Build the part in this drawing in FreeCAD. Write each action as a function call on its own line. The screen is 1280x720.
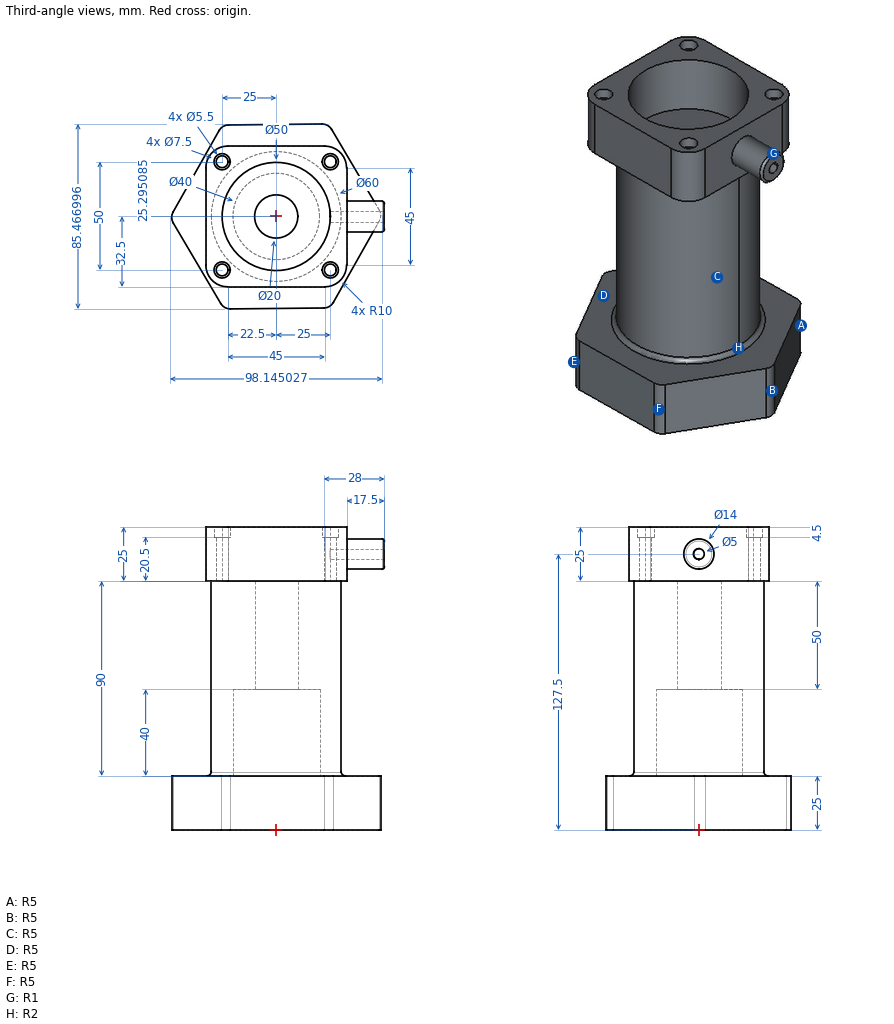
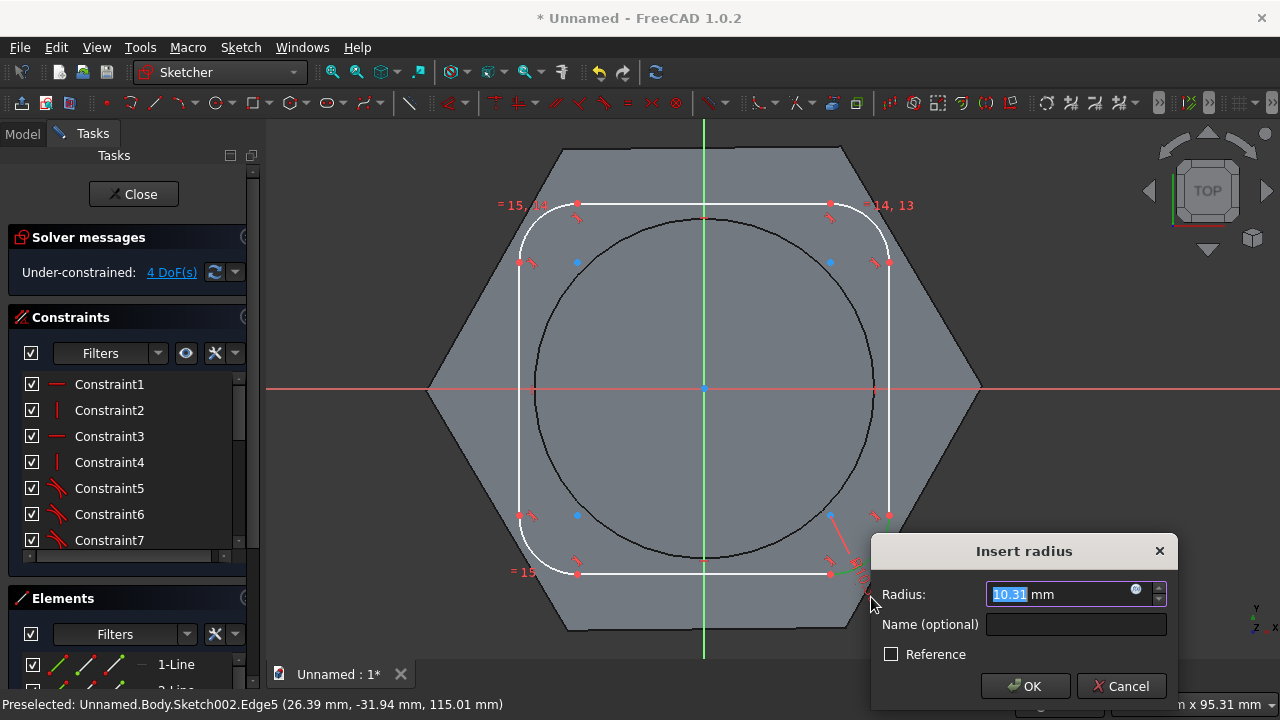
text(10)
key(Return)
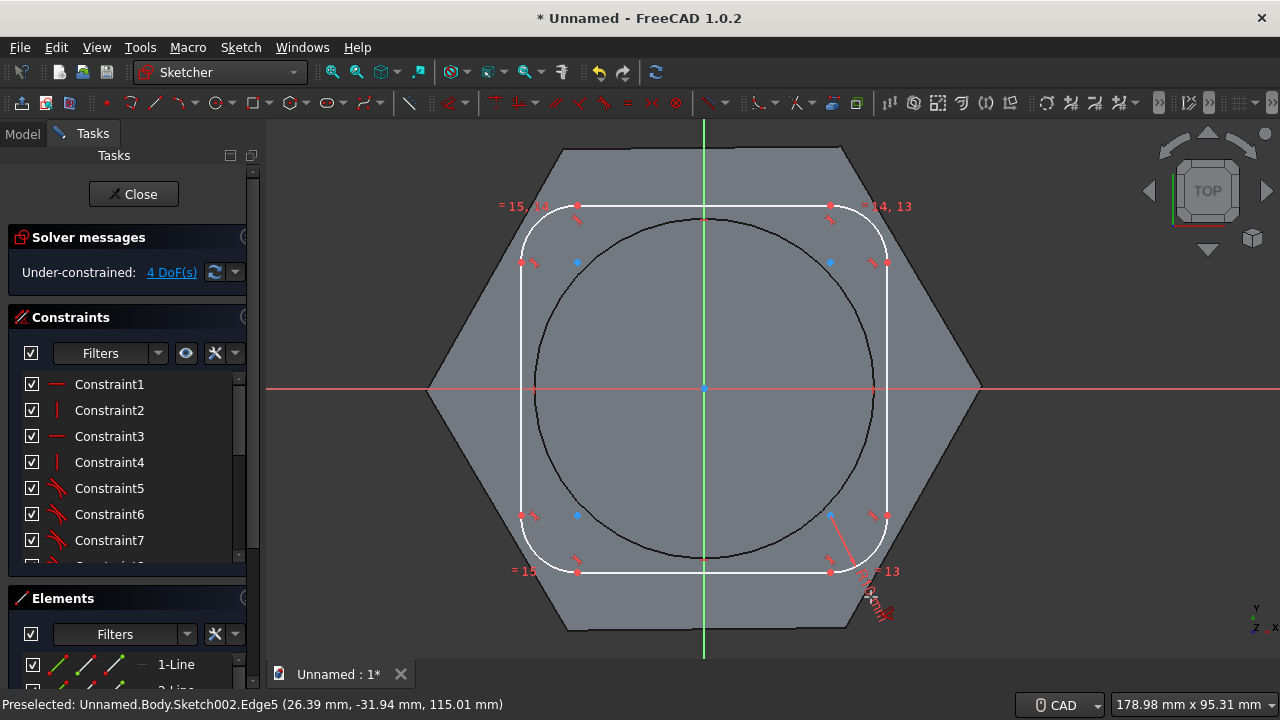
click(654, 573)
click(646, 607)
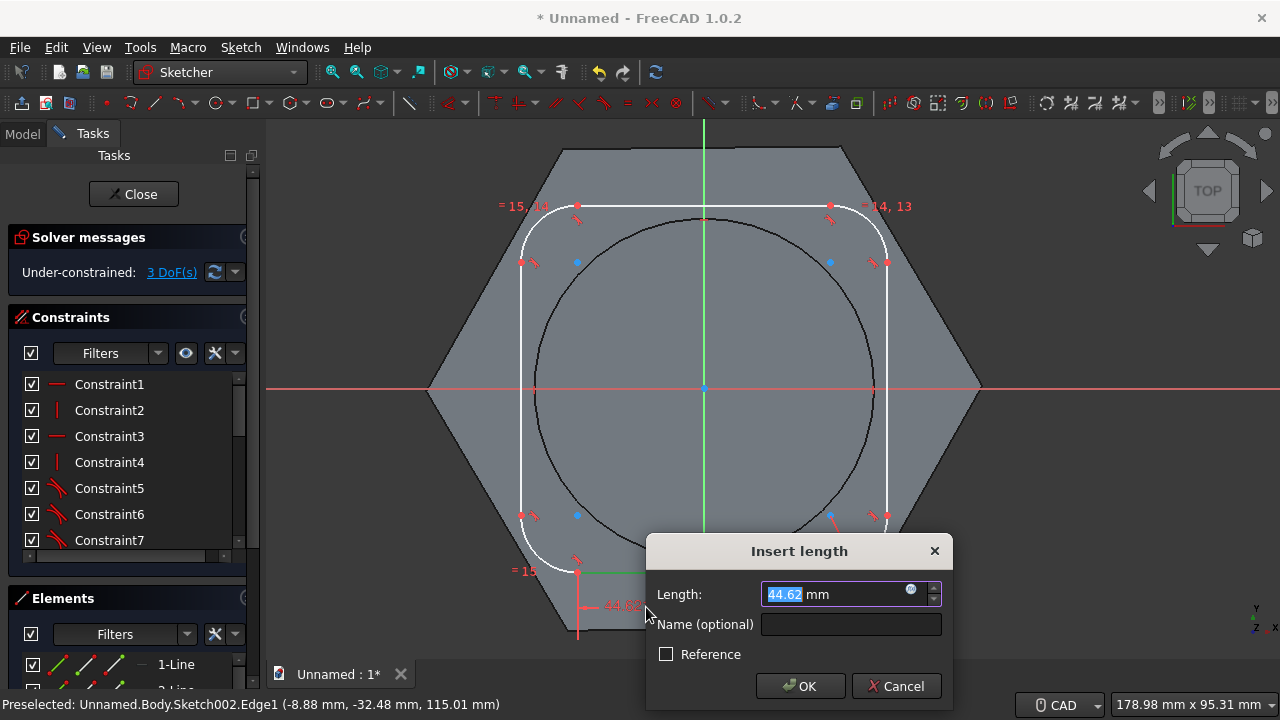
text(45)
key(Return)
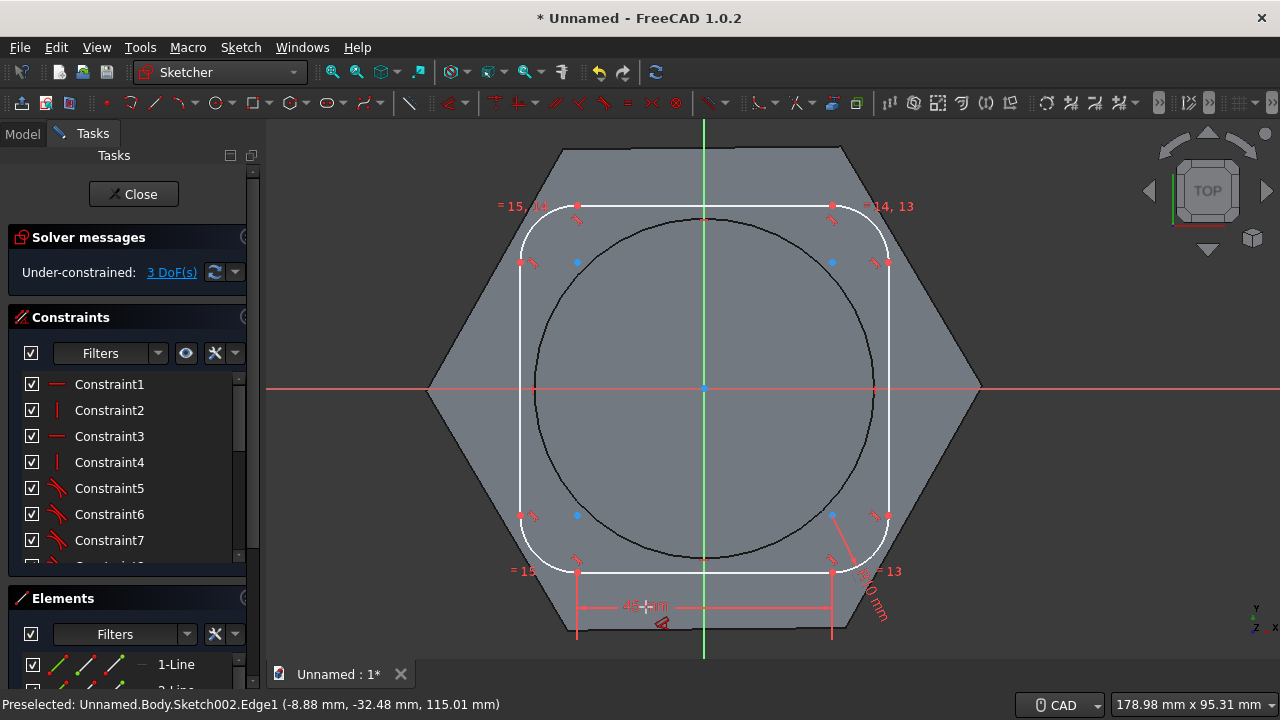
click(889, 440)
click(923, 331)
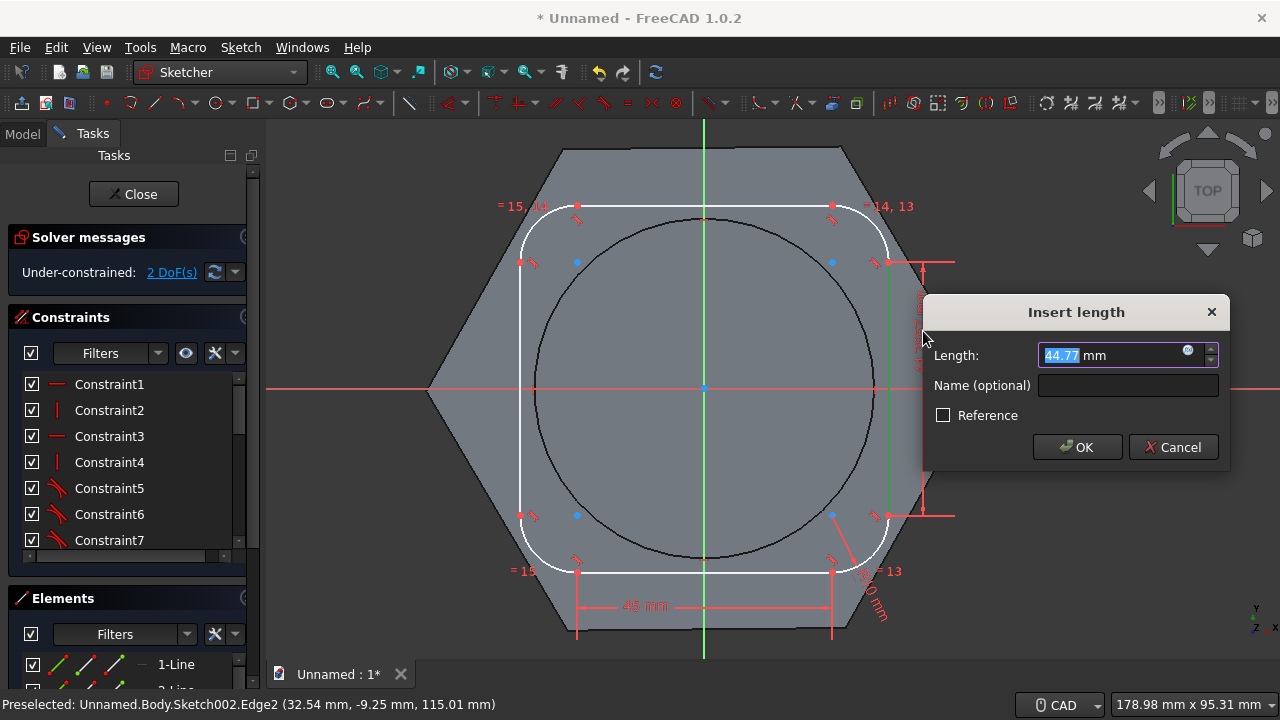
text(45)
key(Return)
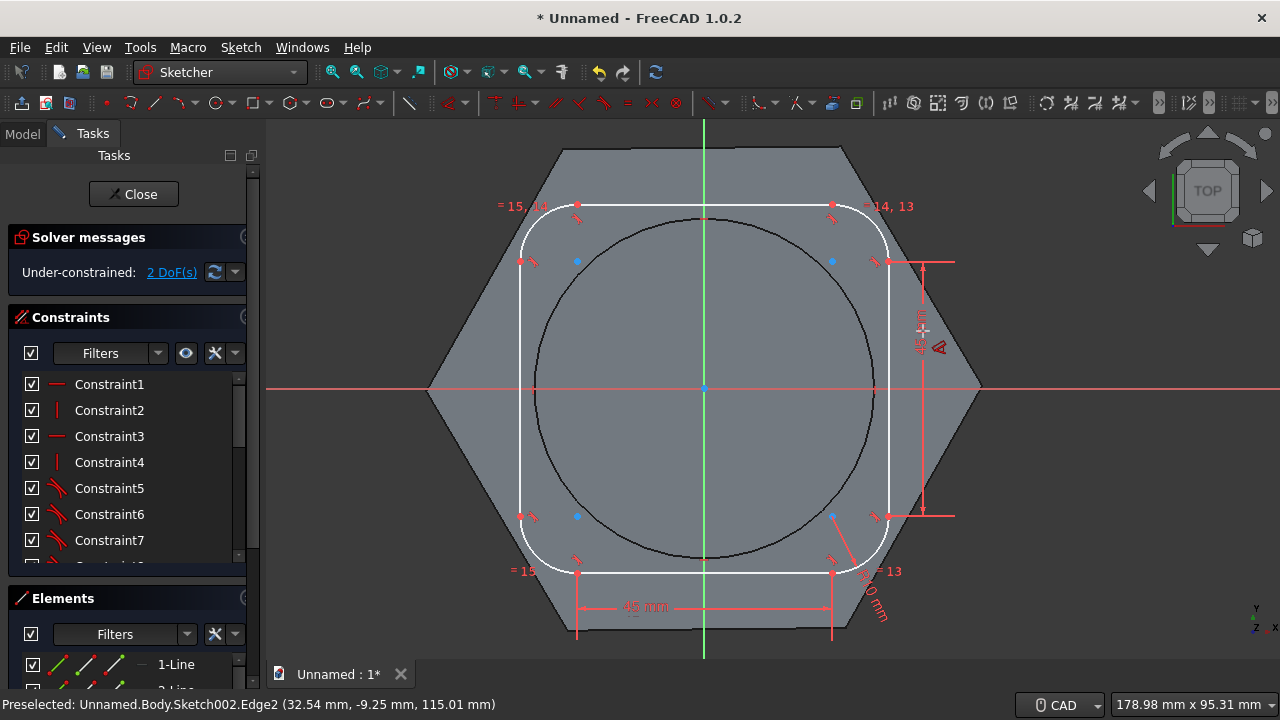
click(577, 573)
click(641, 355)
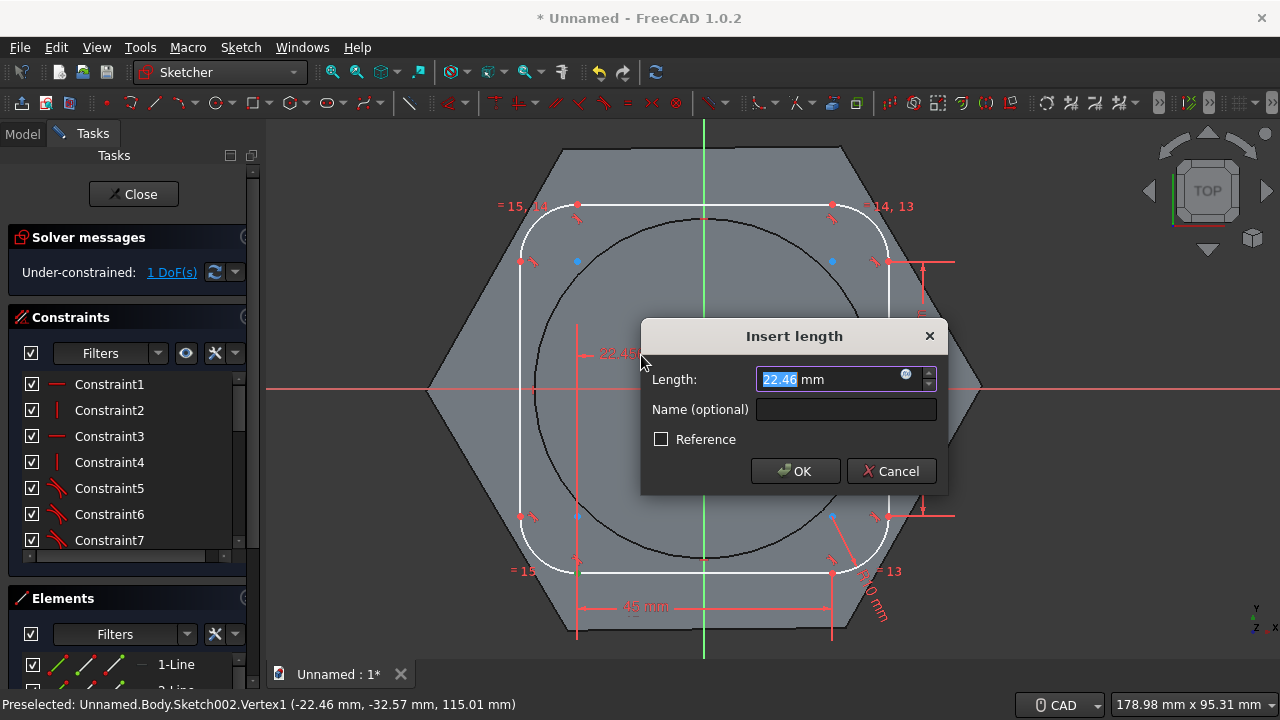
text(22.5)
key(Return)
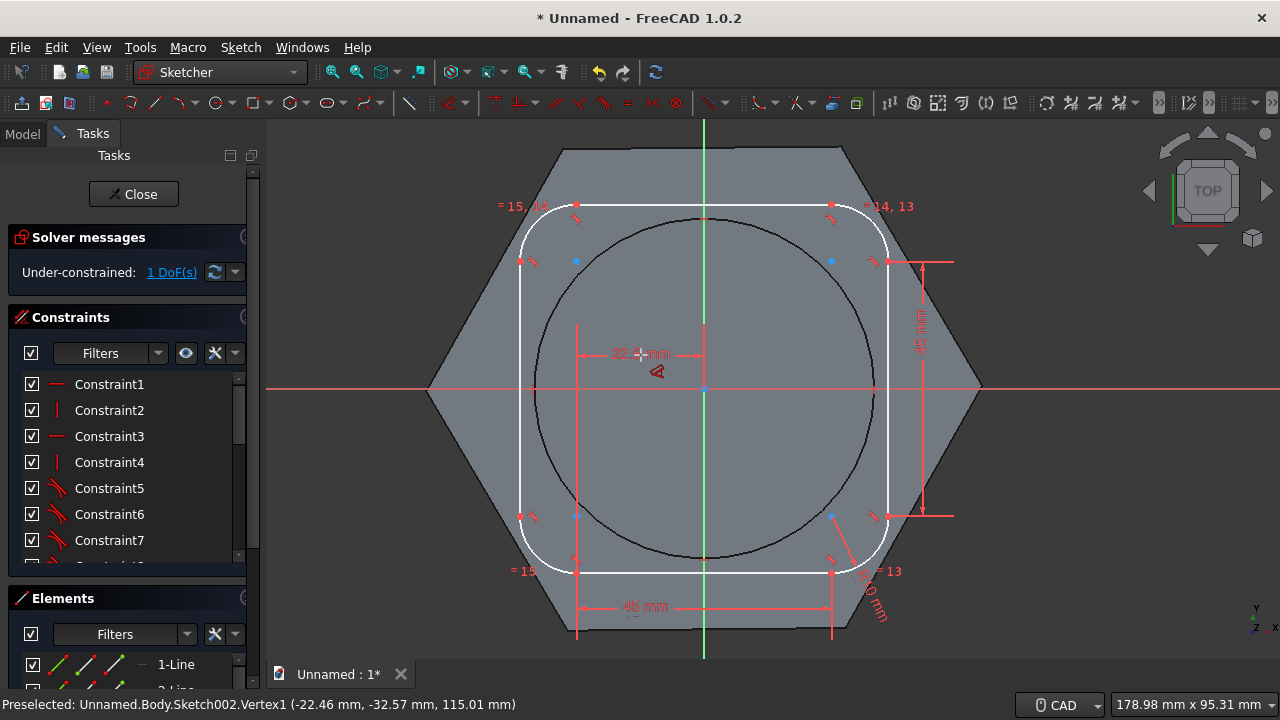
click(577, 573)
click(543, 481)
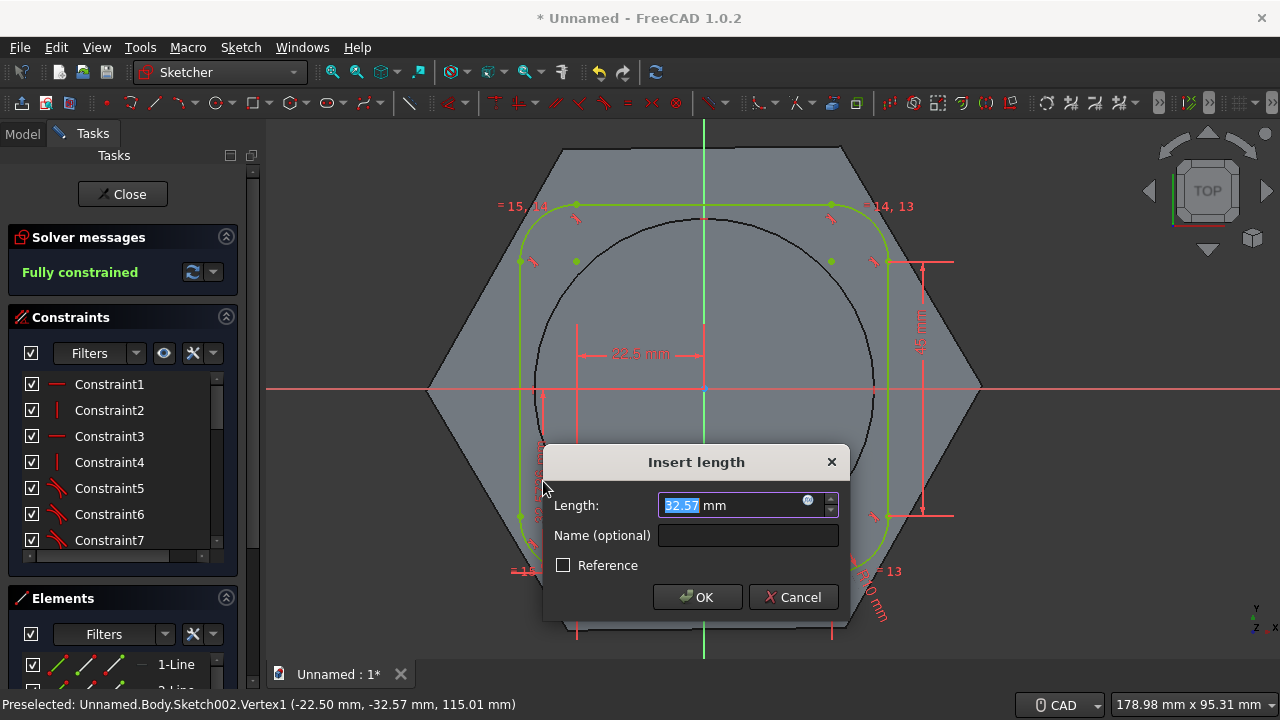
text(32.5)
key(Return)
key(Escape)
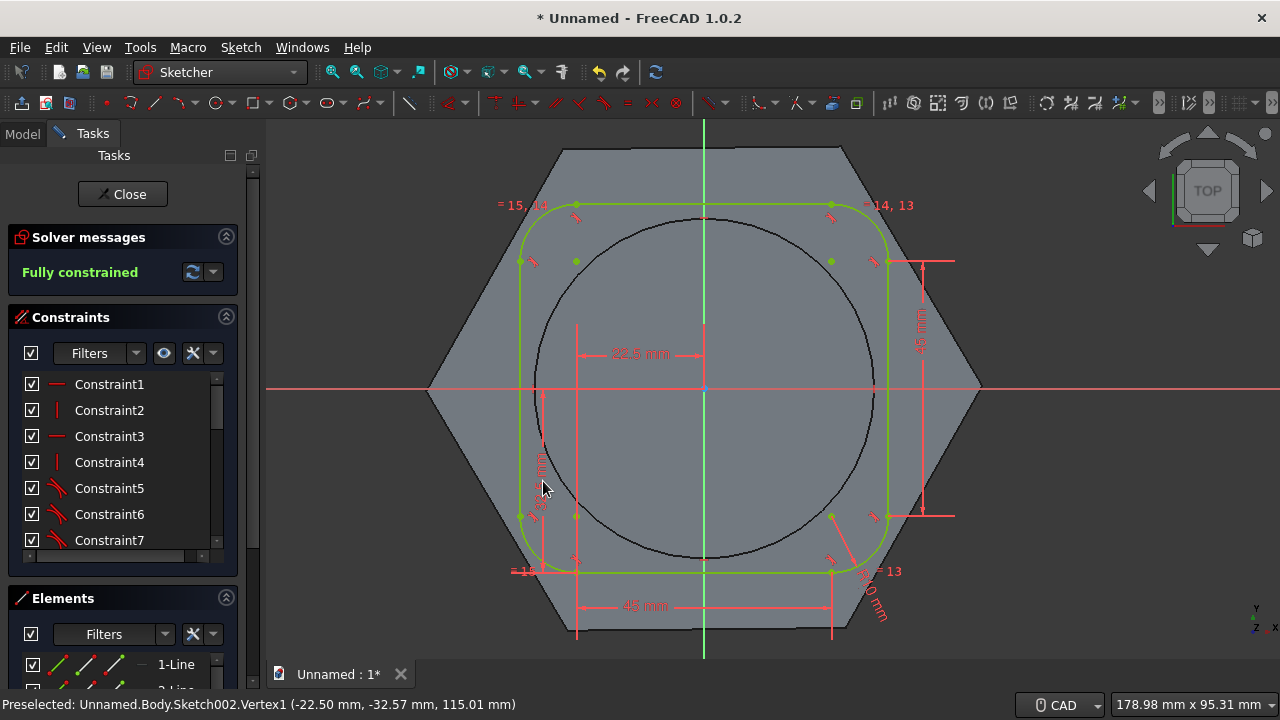
click(123, 194)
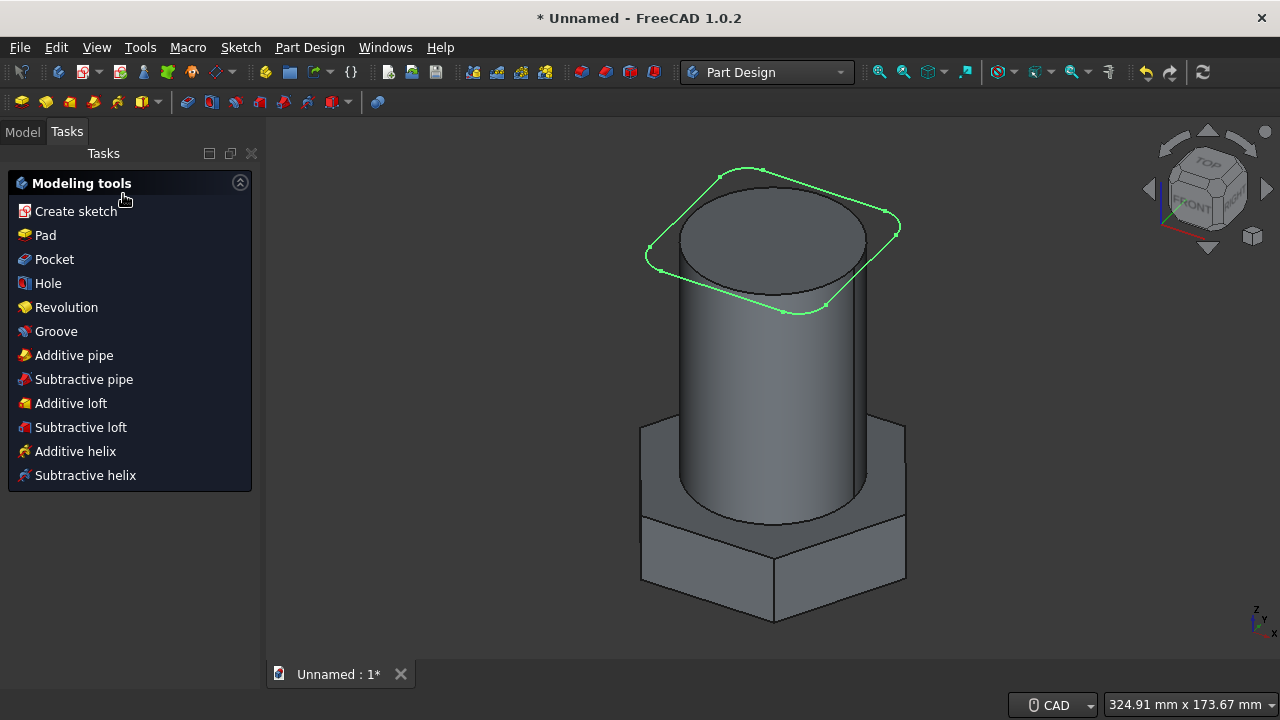
click(22, 102)